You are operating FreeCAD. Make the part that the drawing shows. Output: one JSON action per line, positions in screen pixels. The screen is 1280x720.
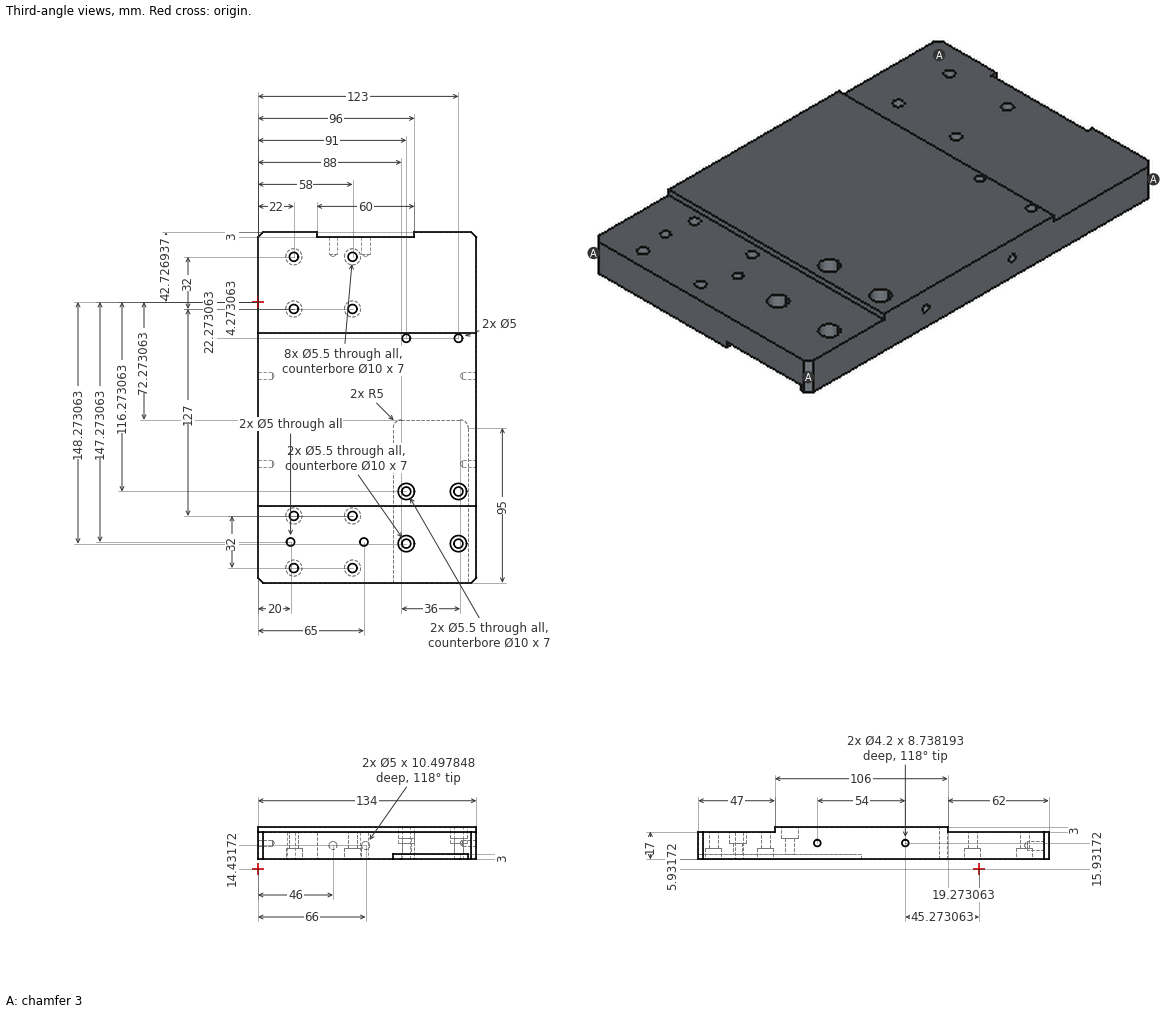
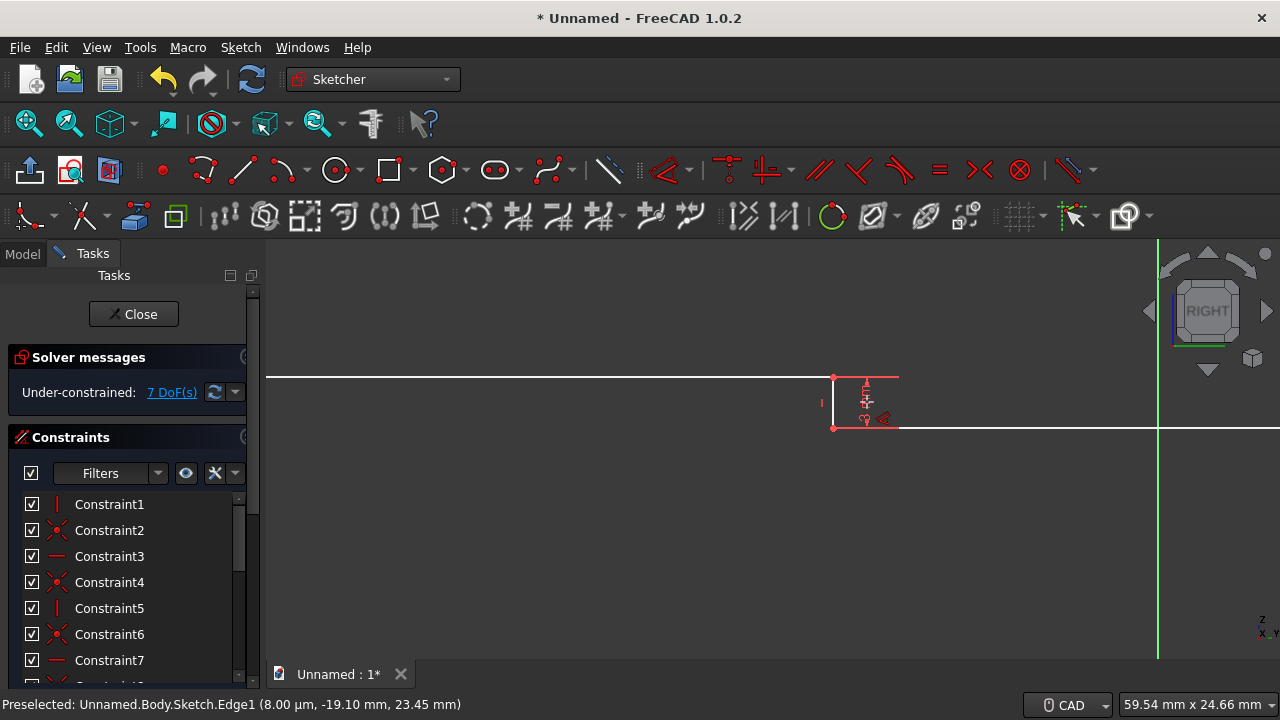
{"action": "scroll", "coordinate": [833, 421], "scroll_direction": "down", "scroll_amount": 9}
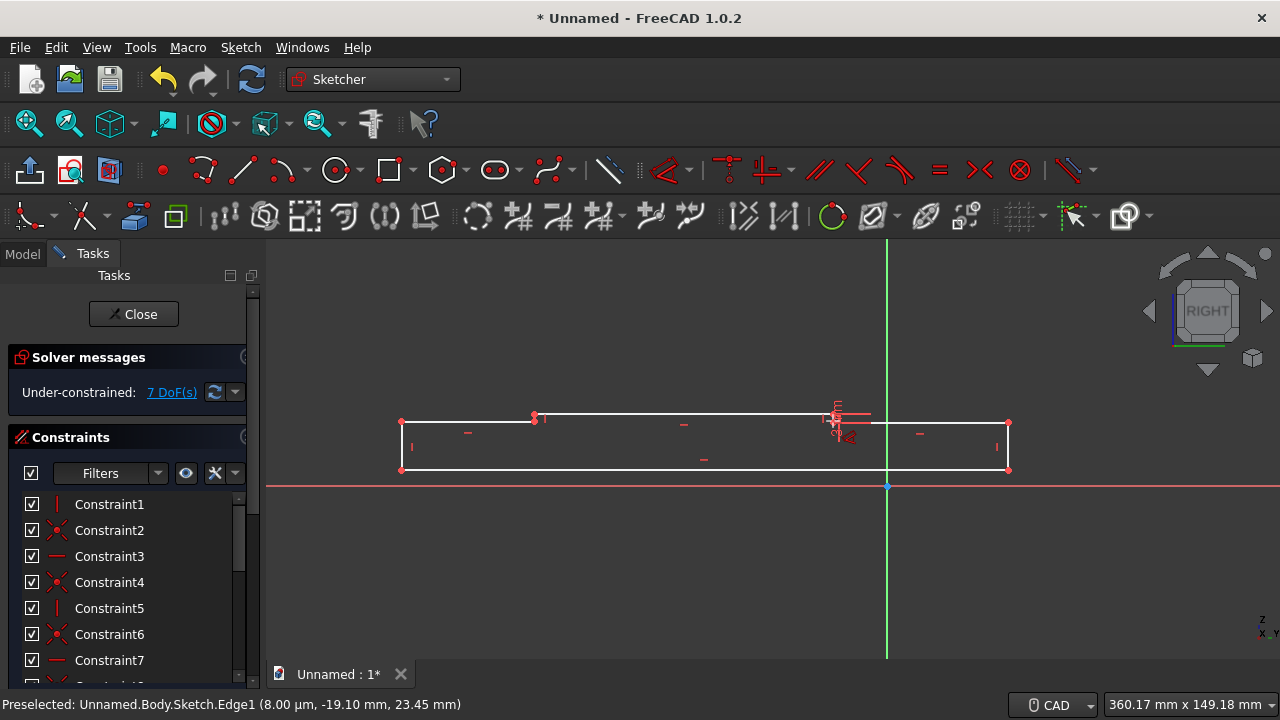
{"action": "scroll", "coordinate": [535, 416], "scroll_direction": "up", "scroll_amount": 9}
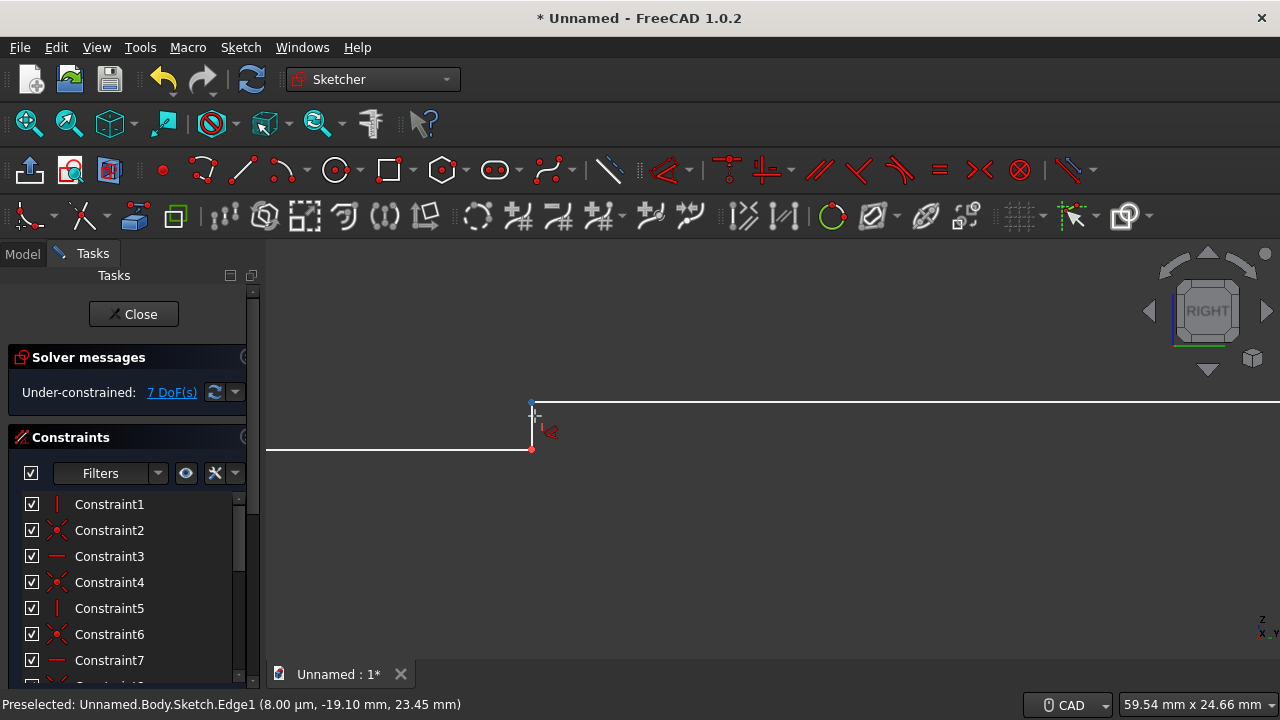
{"action": "left_click", "coordinate": [532, 417]}
{"action": "left_click", "coordinate": [498, 426]}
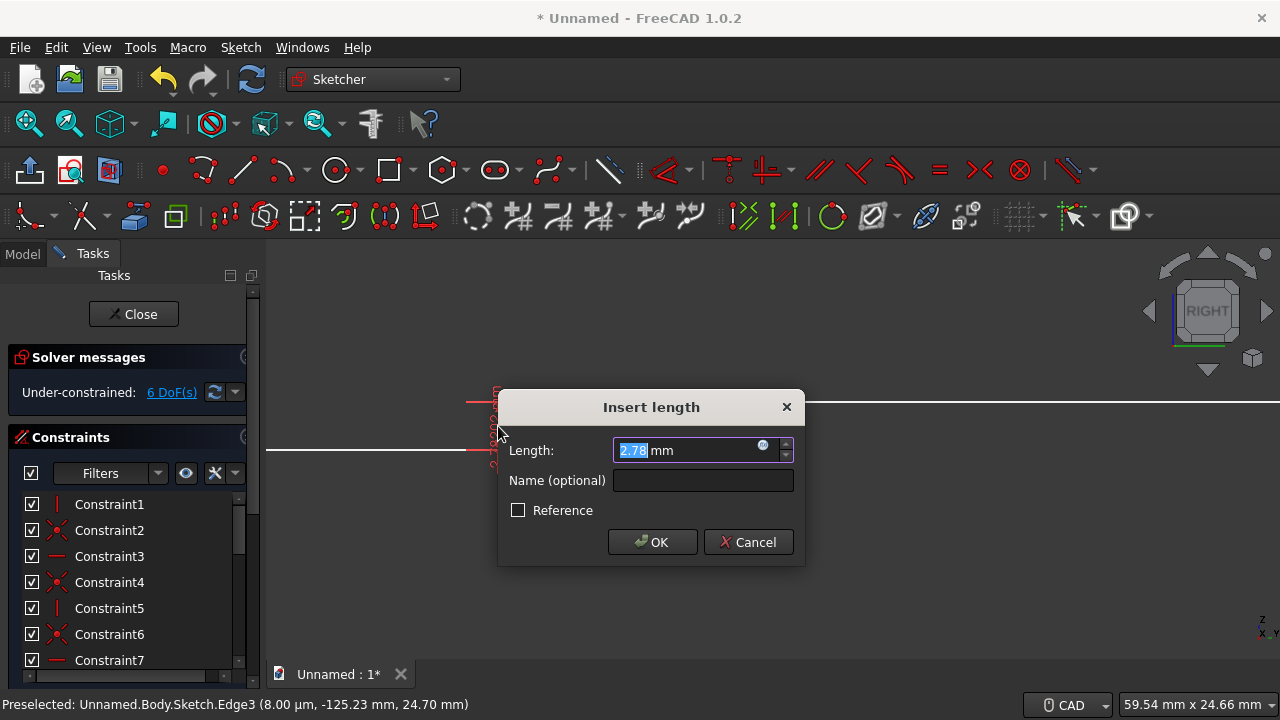
{"action": "type", "text": "3"}
{"action": "key", "text": "Return"}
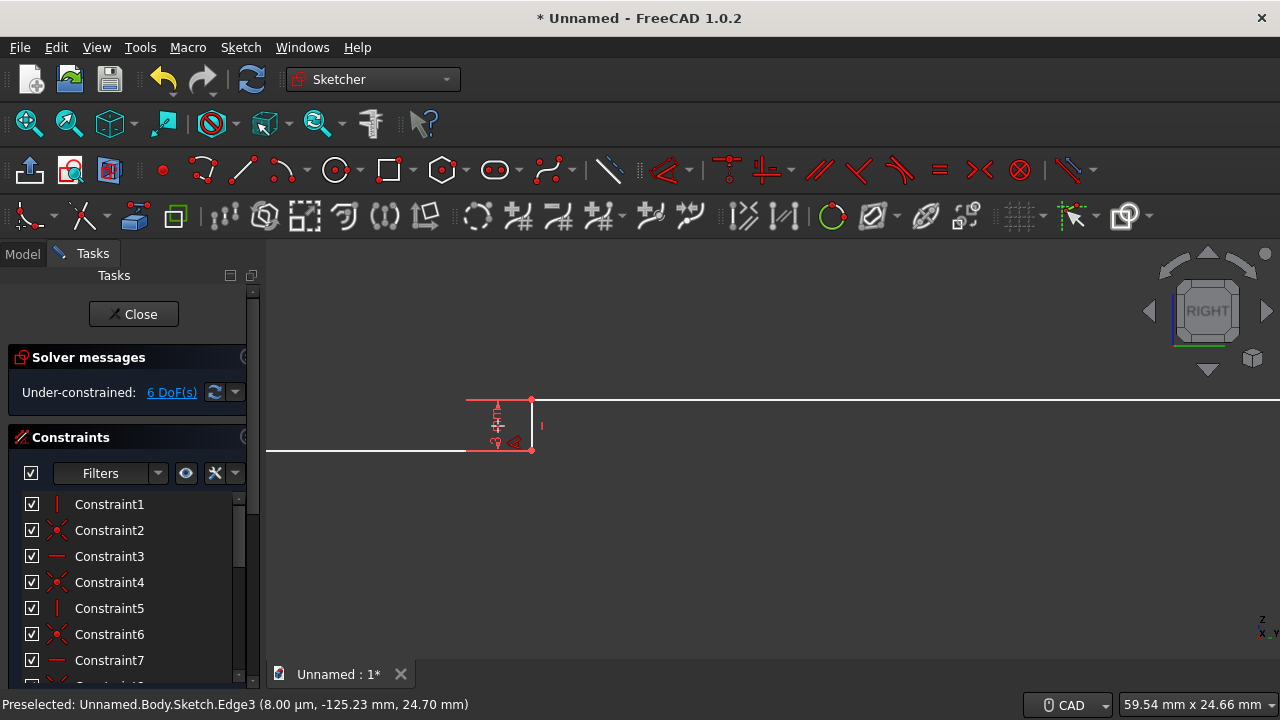
{"action": "scroll", "coordinate": [535, 416], "scroll_direction": "down", "scroll_amount": 9}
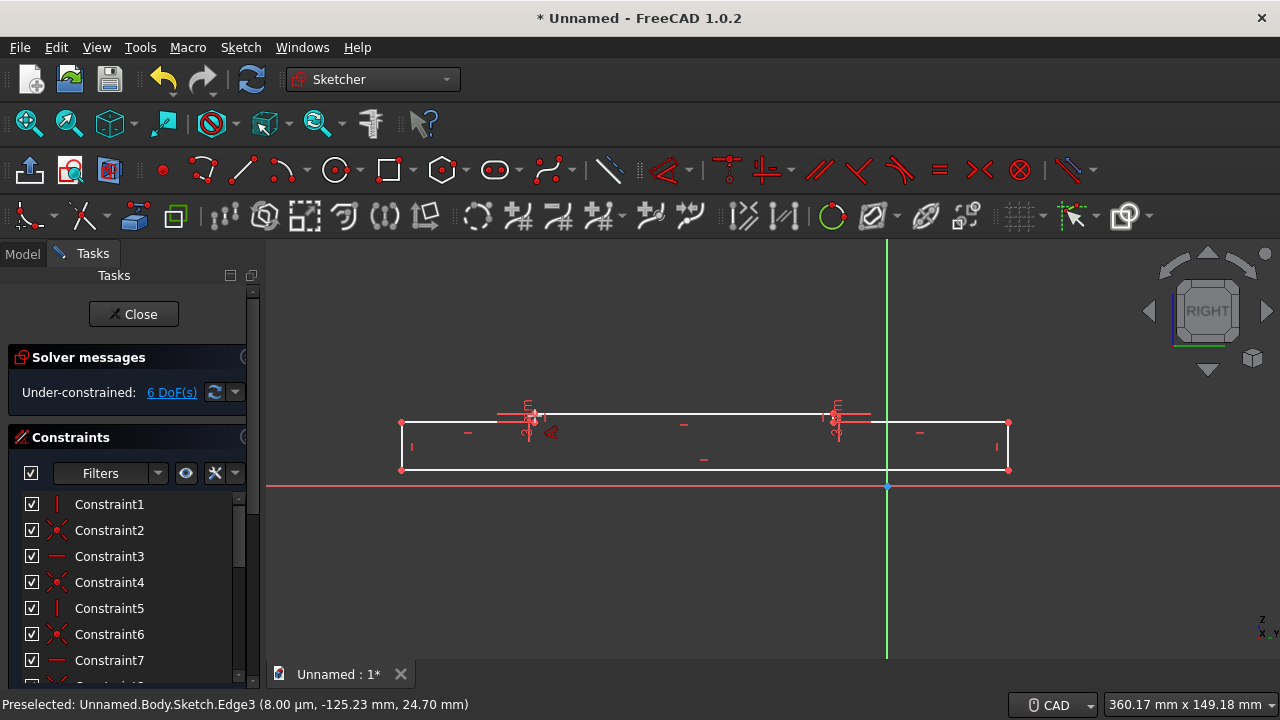
{"action": "left_click", "coordinate": [508, 422]}
{"action": "left_click", "coordinate": [468, 388]}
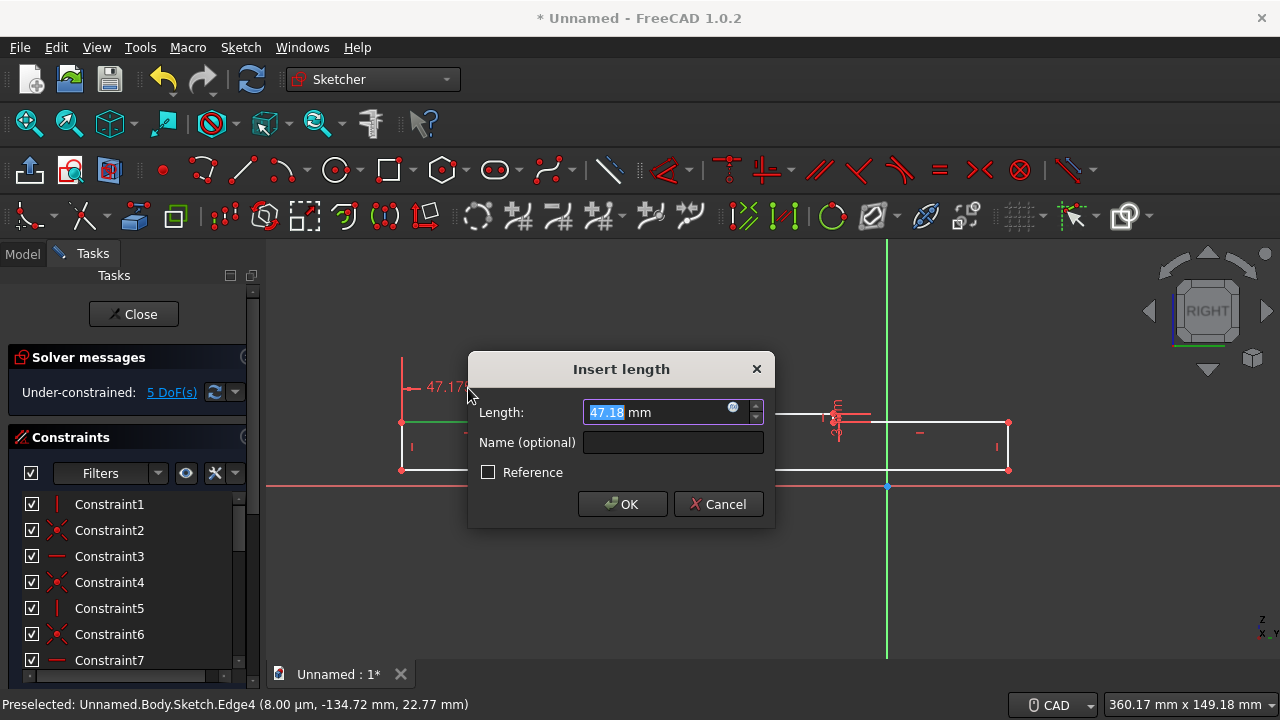
{"action": "type", "text": "47"}
{"action": "key", "text": "Return"}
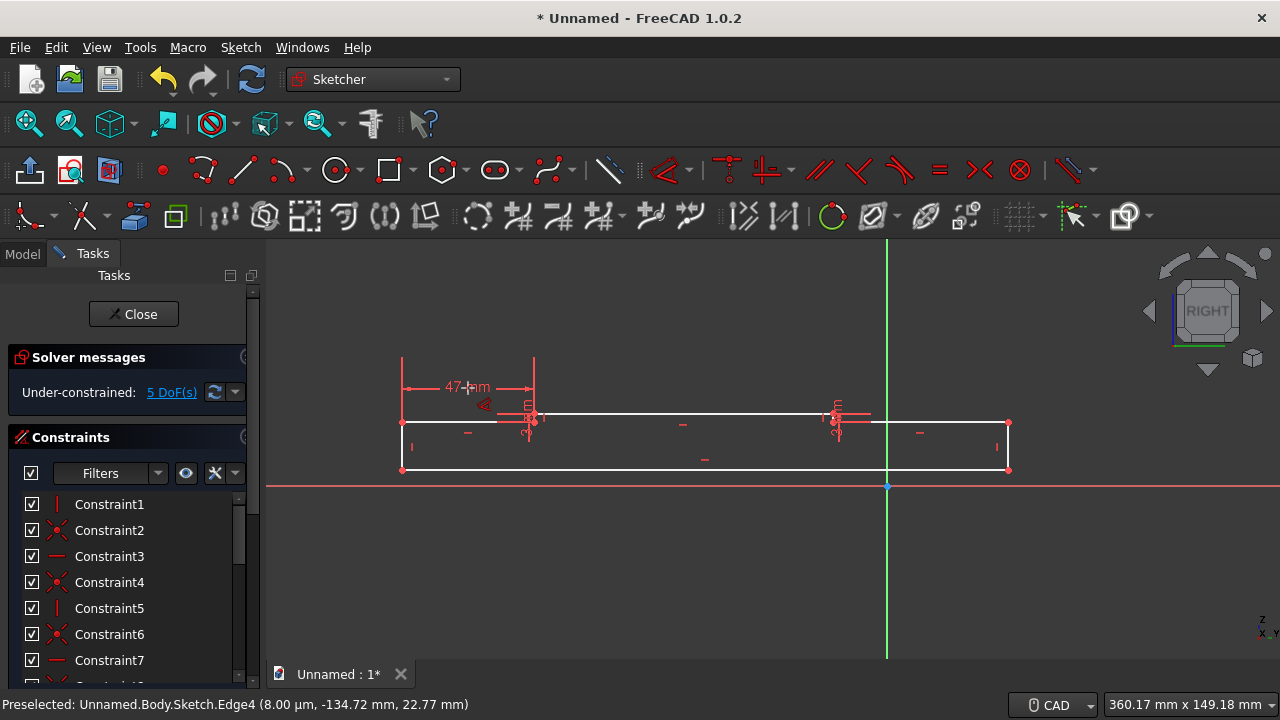
{"action": "left_click", "coordinate": [402, 437]}
{"action": "left_click", "coordinate": [368, 446]}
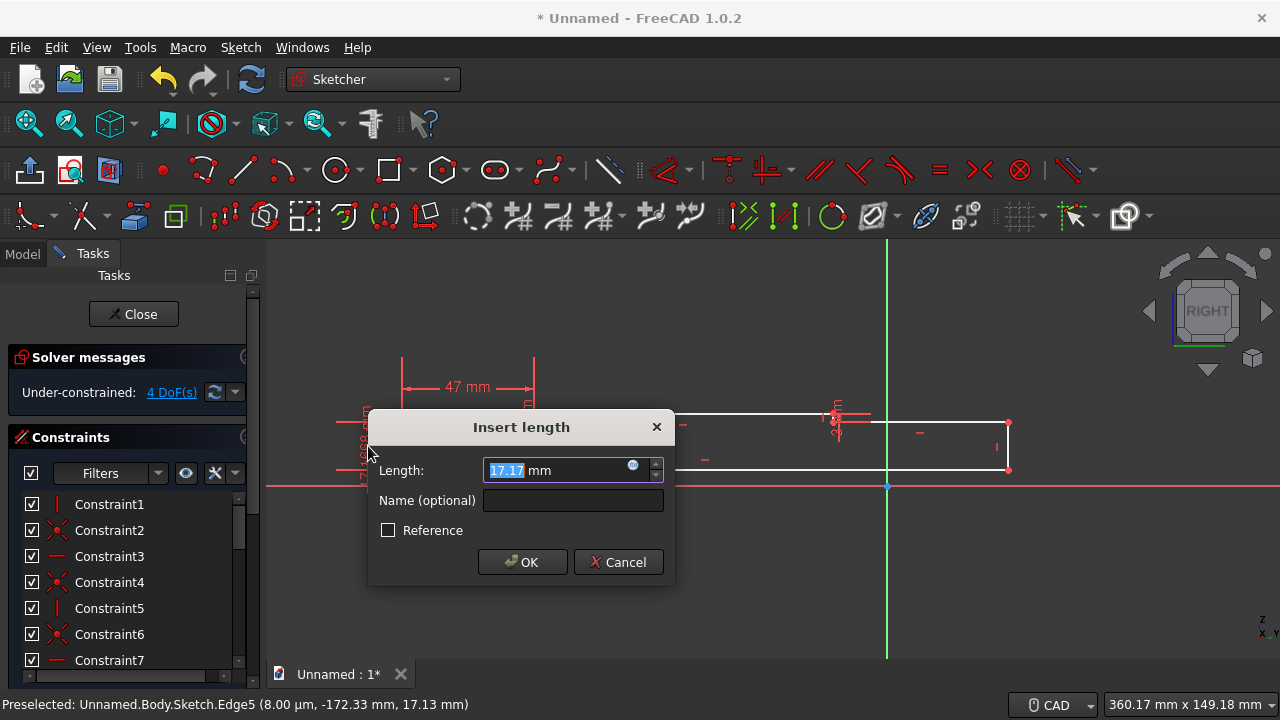
{"action": "type", "text": "17"}
{"action": "key", "text": "Return"}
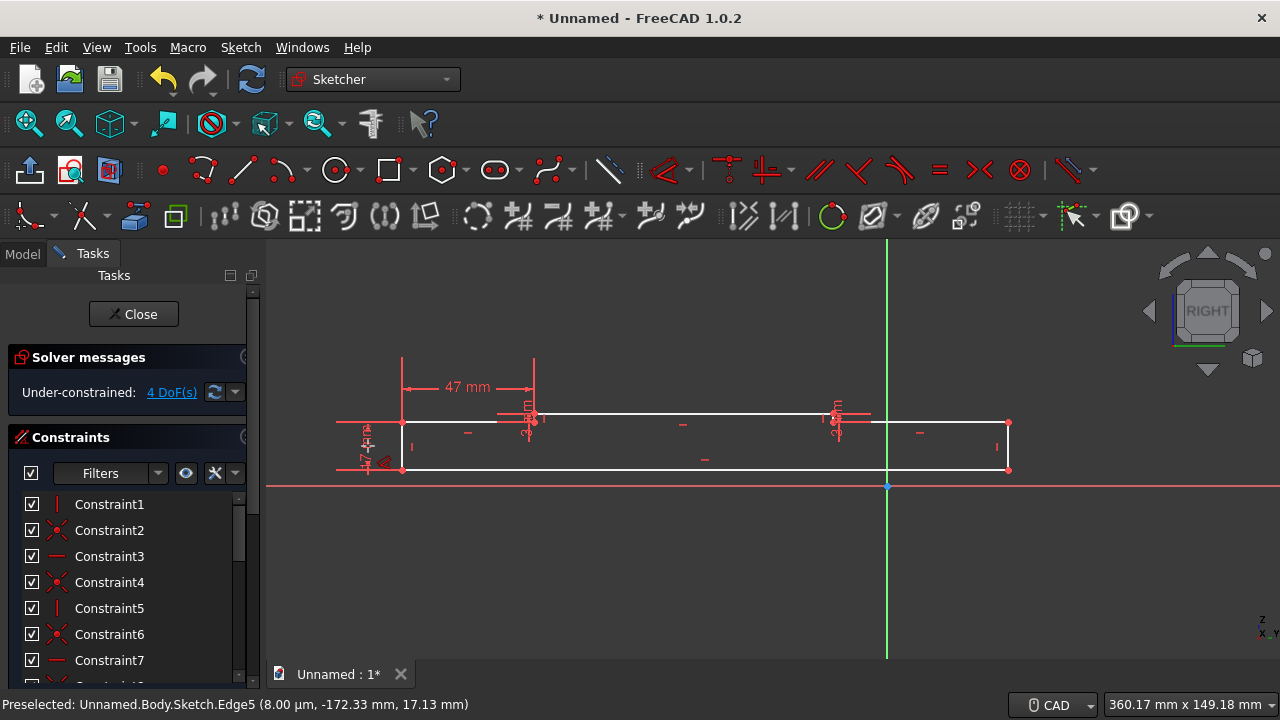
{"action": "left_click", "coordinate": [956, 422]}
{"action": "left_click", "coordinate": [921, 388]}